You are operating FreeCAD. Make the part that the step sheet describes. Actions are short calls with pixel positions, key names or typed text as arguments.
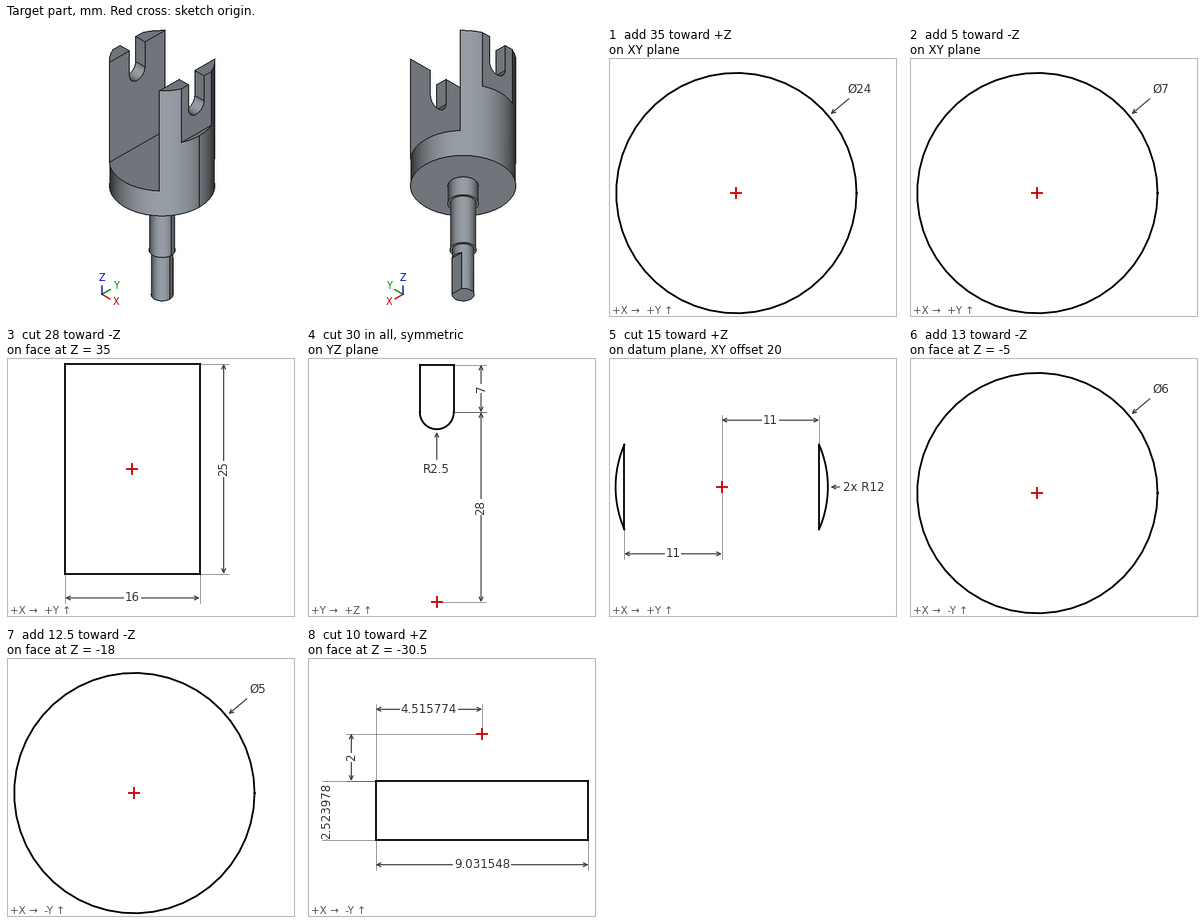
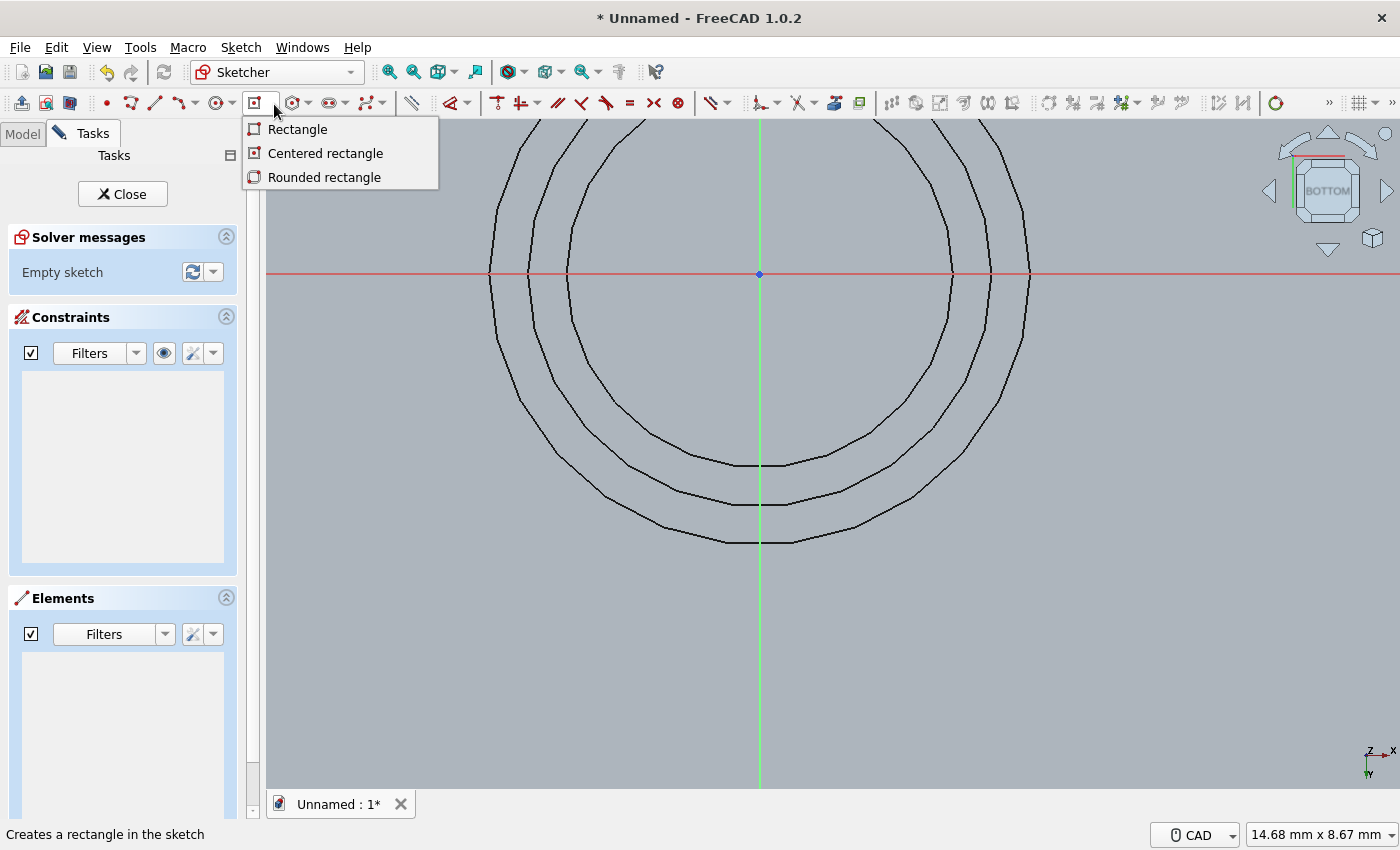
click(340, 129)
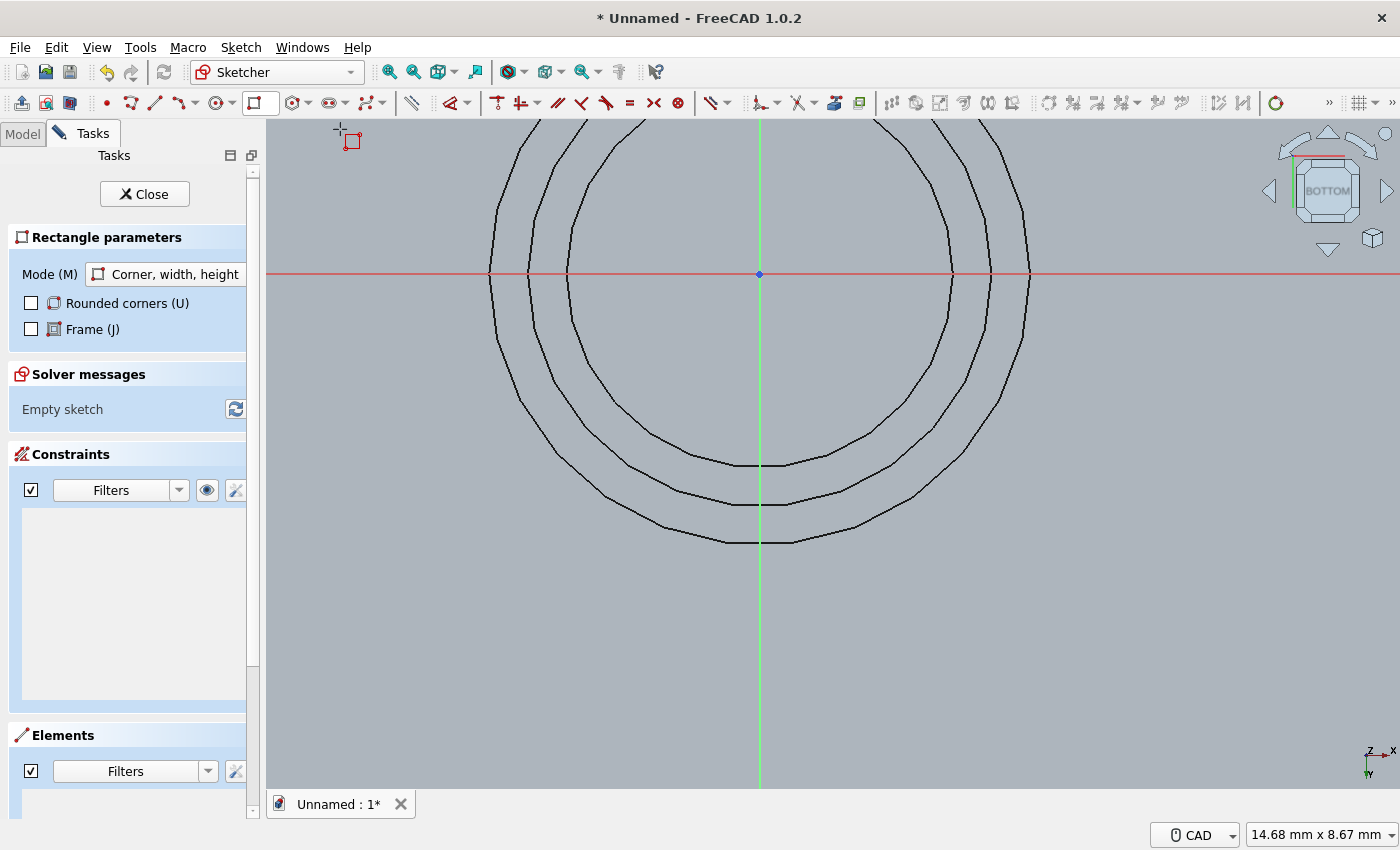
click(411, 429)
click(1109, 624)
key(Escape)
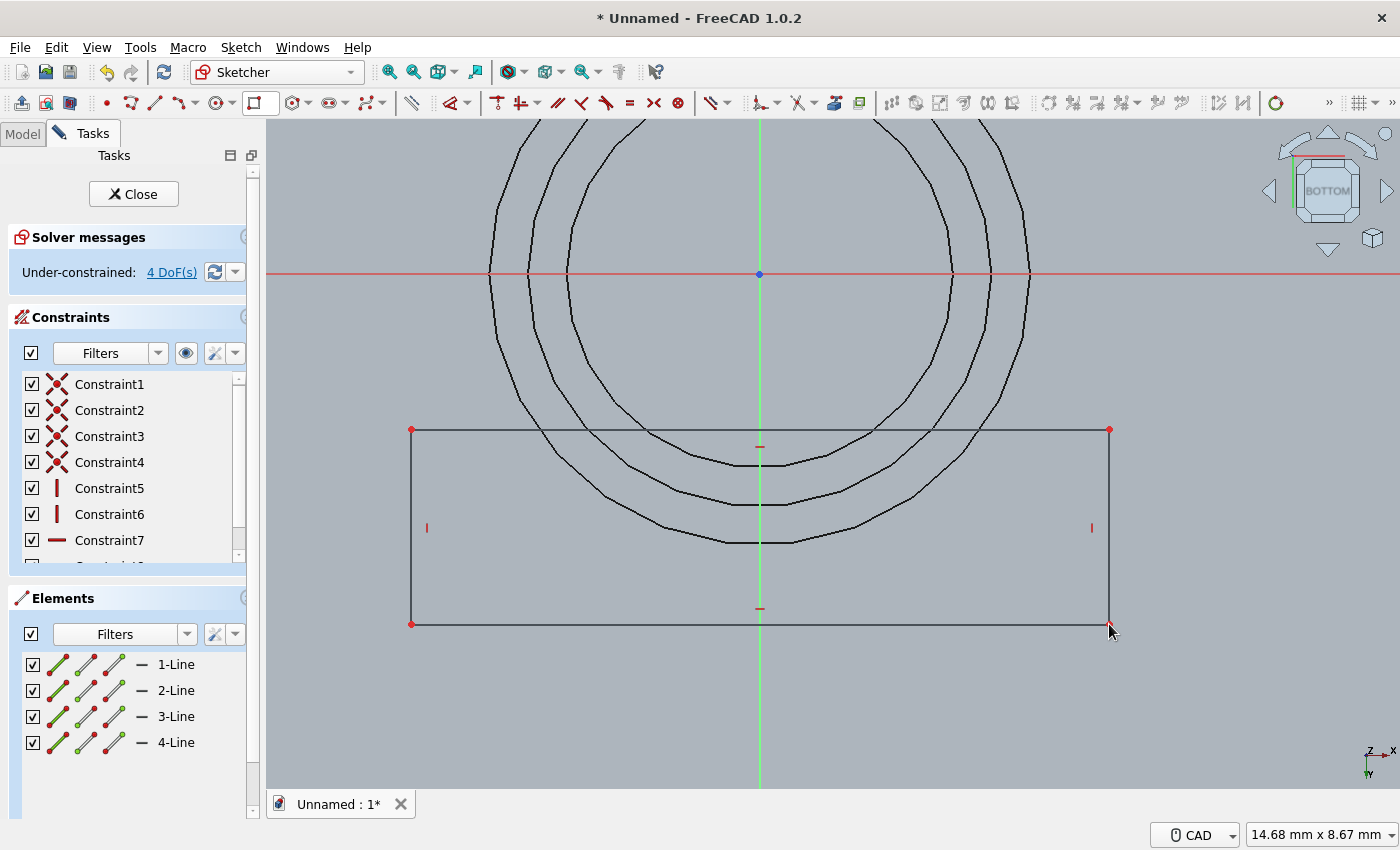
key(d)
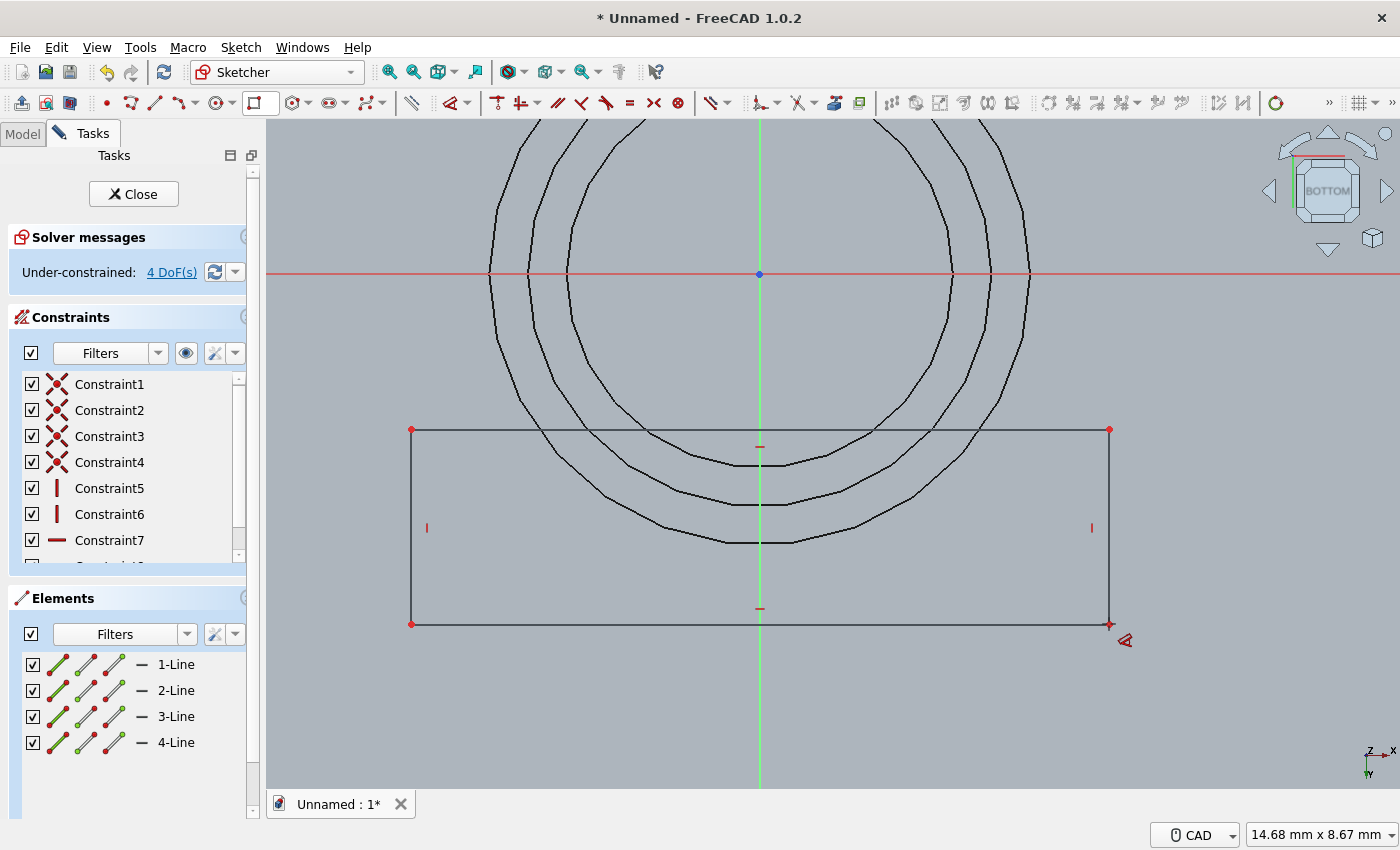
click(411, 430)
click(377, 352)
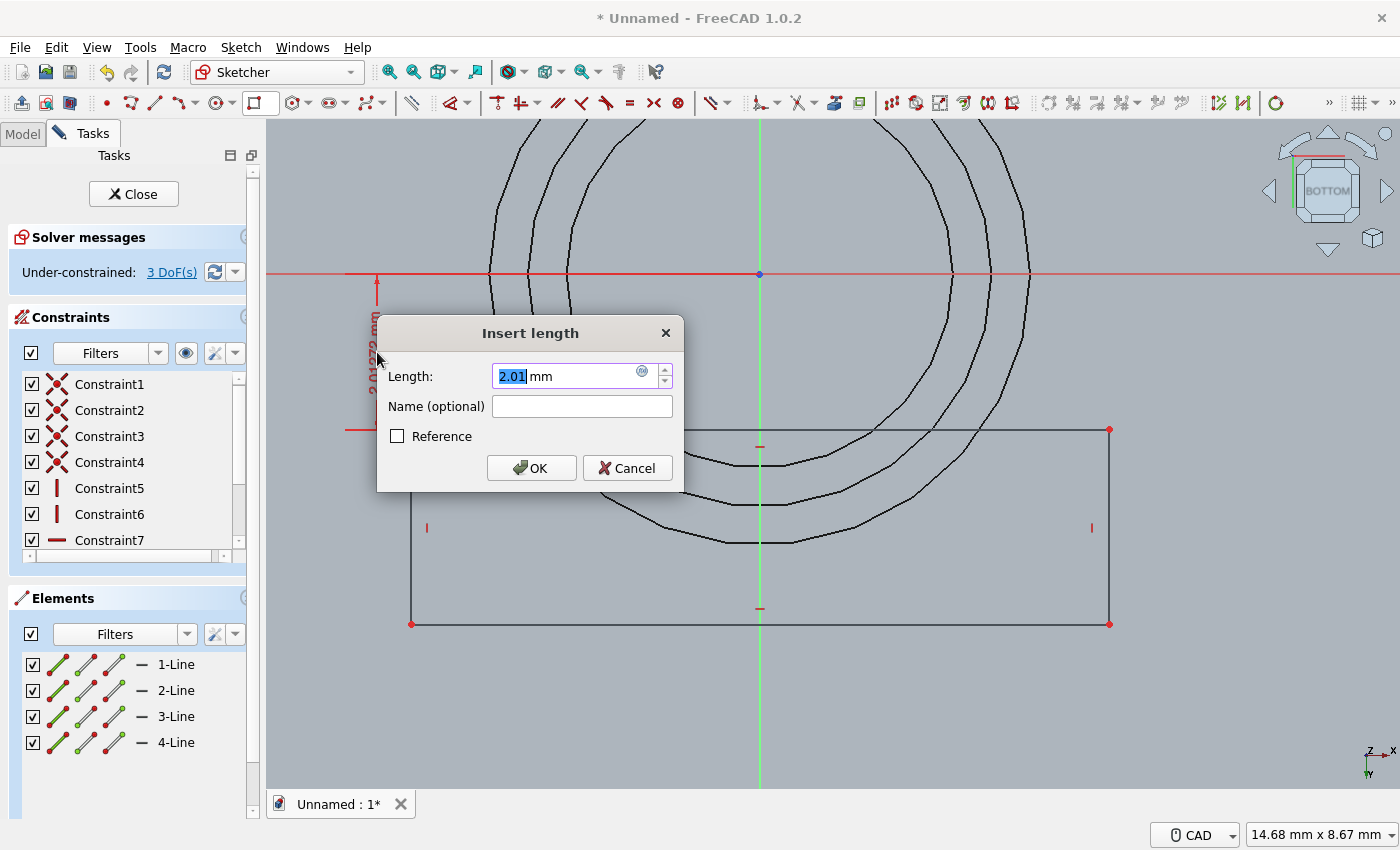
text(2)
key(Return)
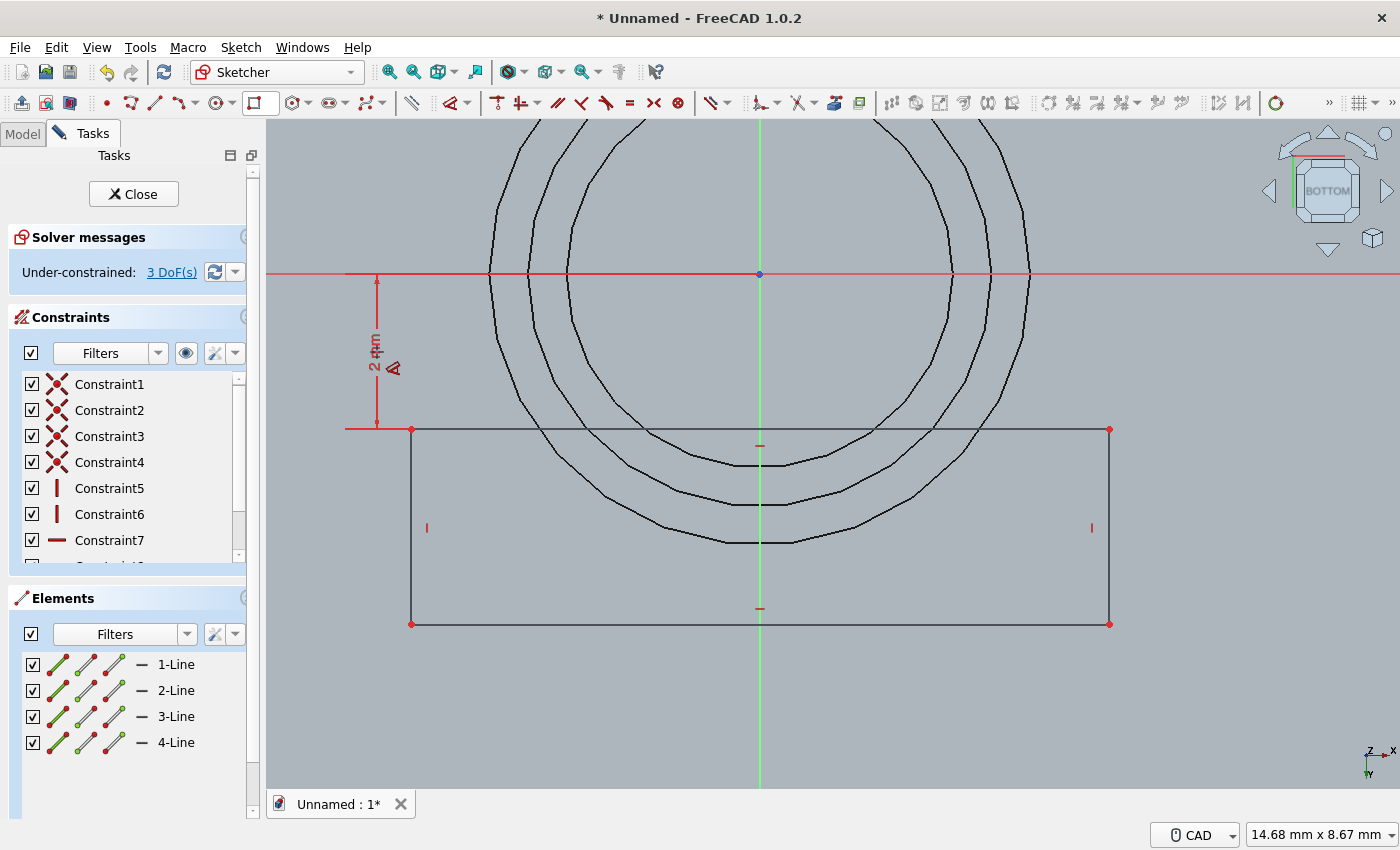
click(411, 488)
click(377, 527)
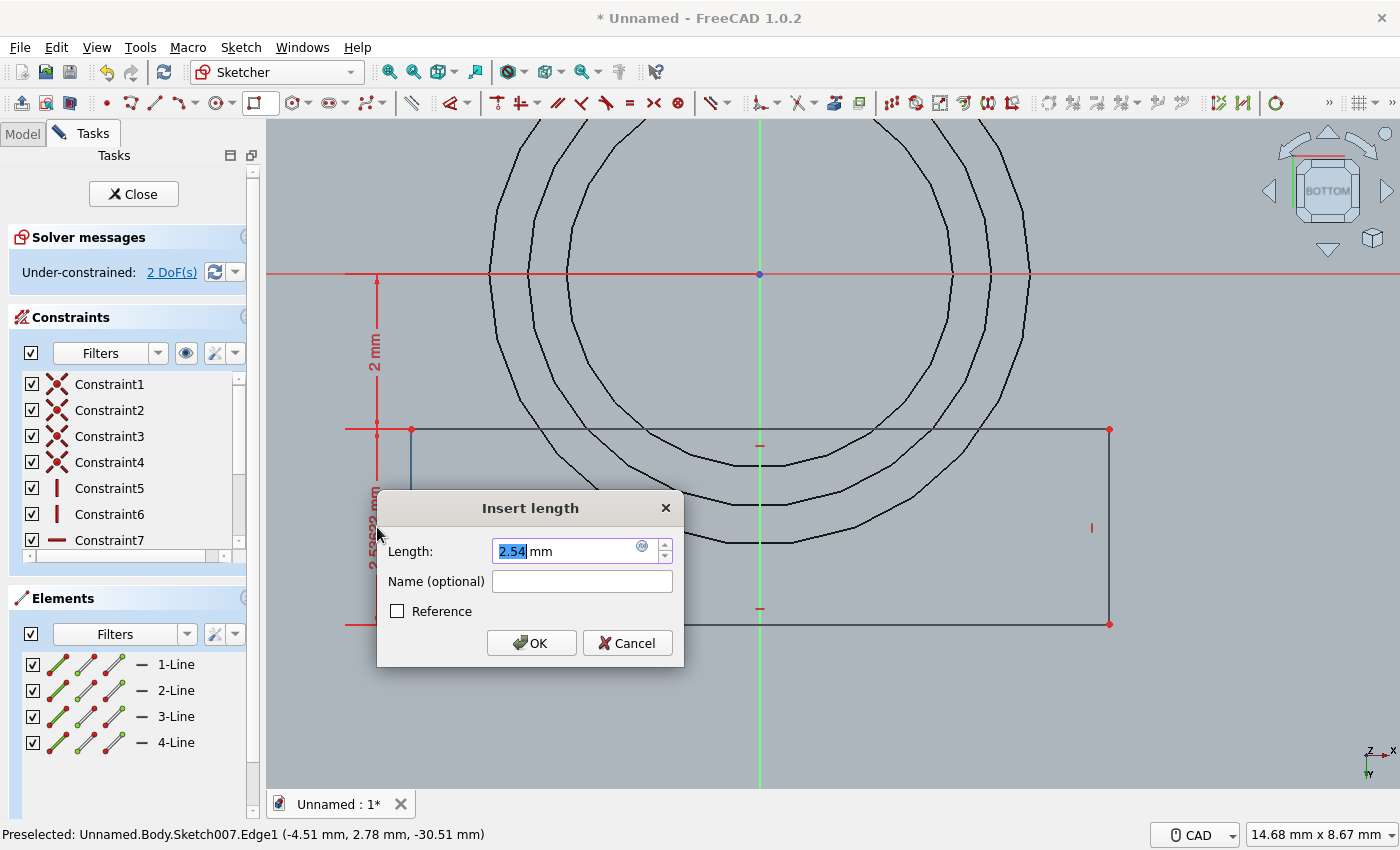
text(2.523978)
key(Return)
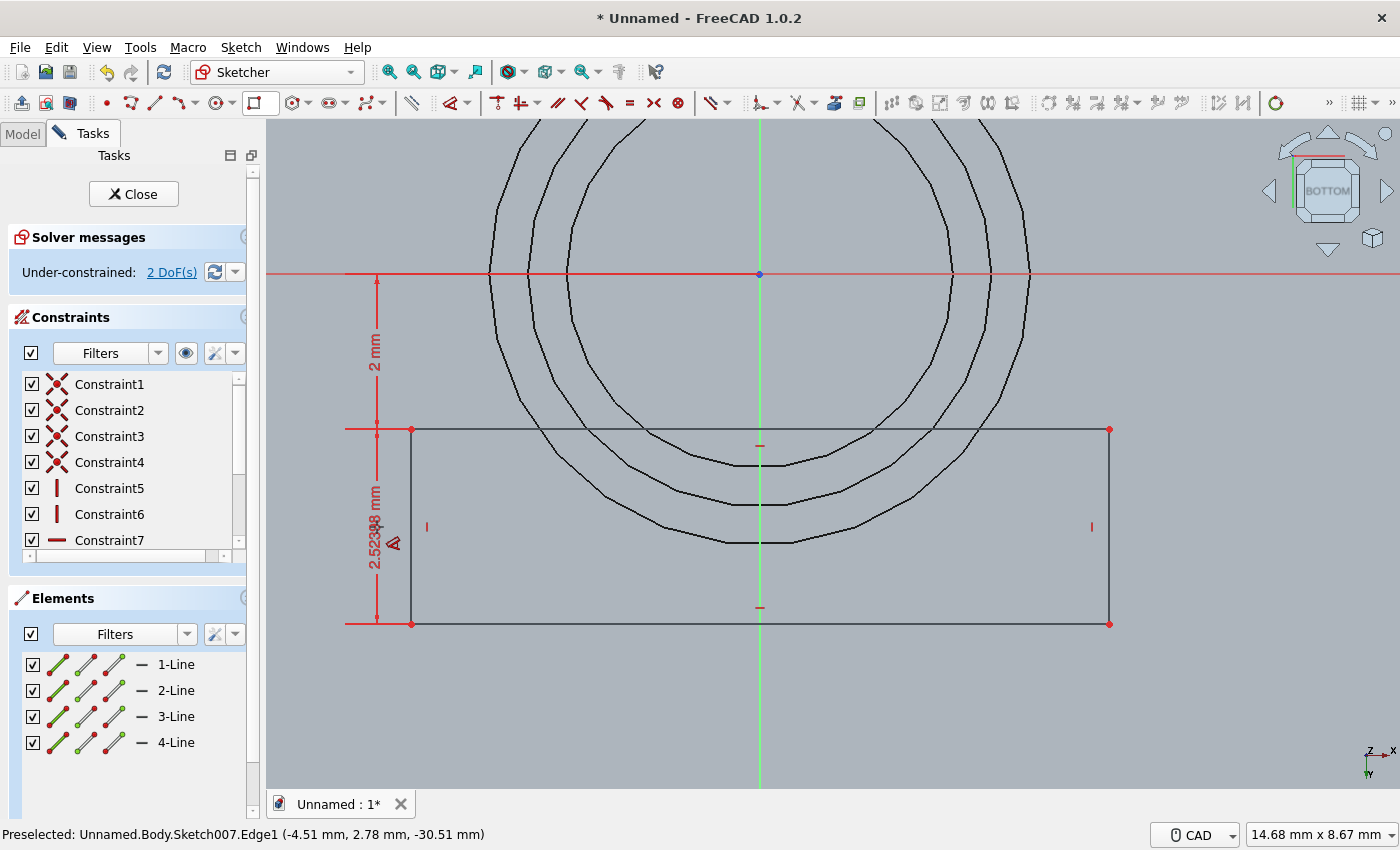
click(620, 624)
click(599, 658)